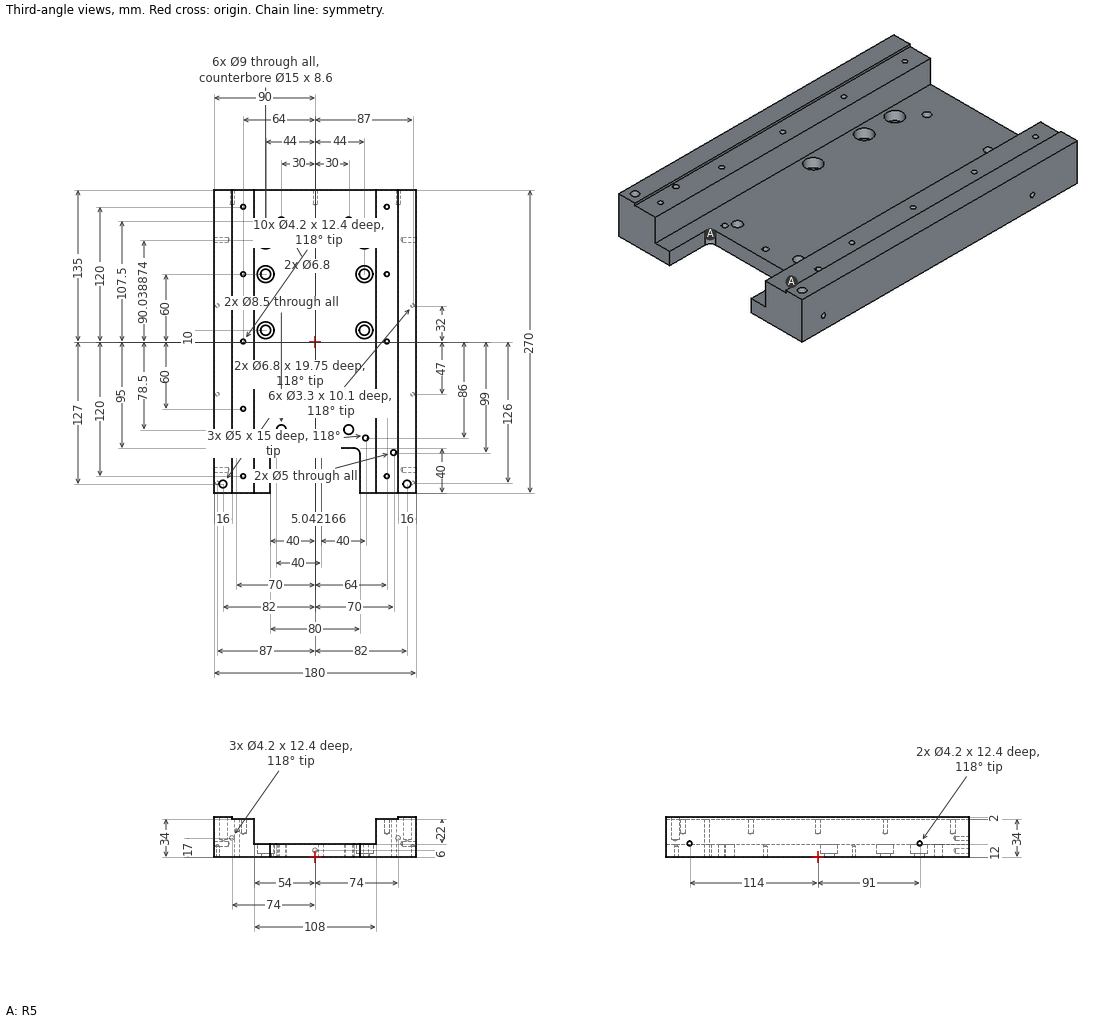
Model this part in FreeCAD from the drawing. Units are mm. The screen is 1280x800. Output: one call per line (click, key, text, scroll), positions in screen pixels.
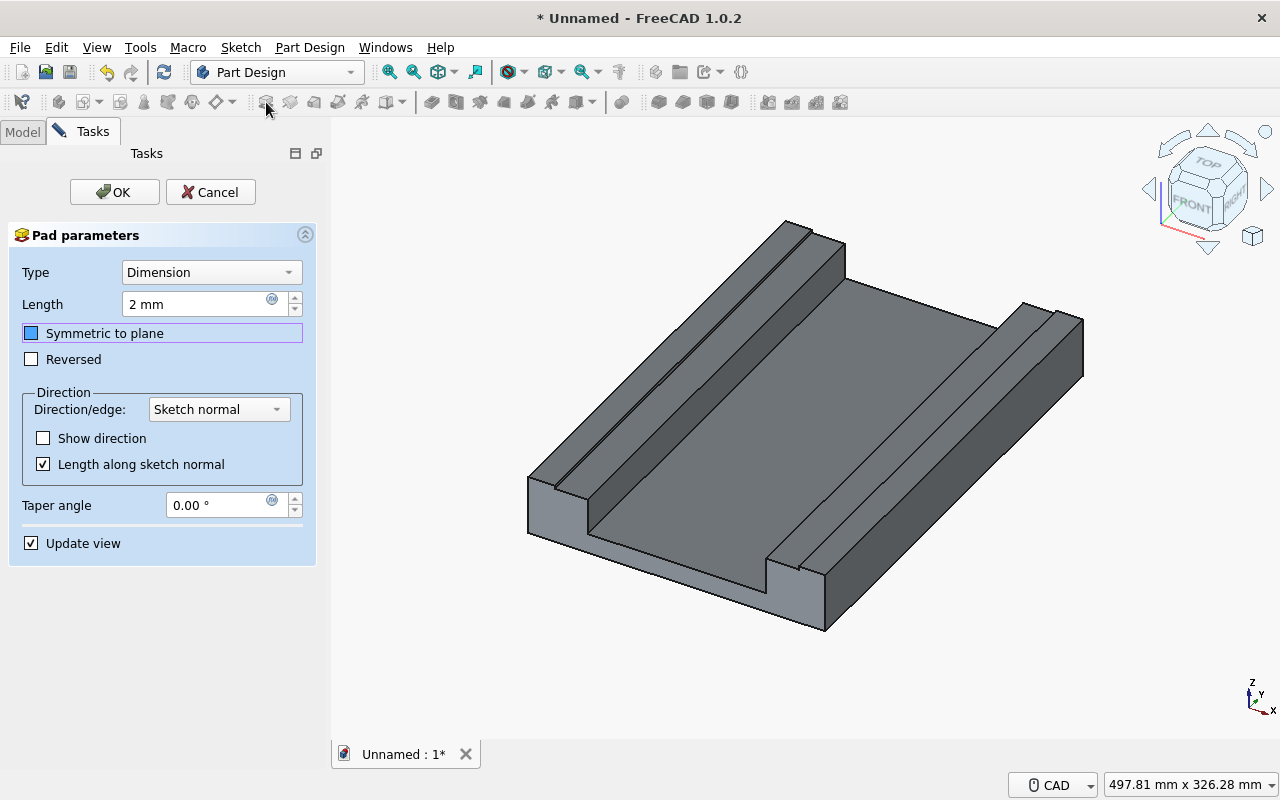
click(115, 192)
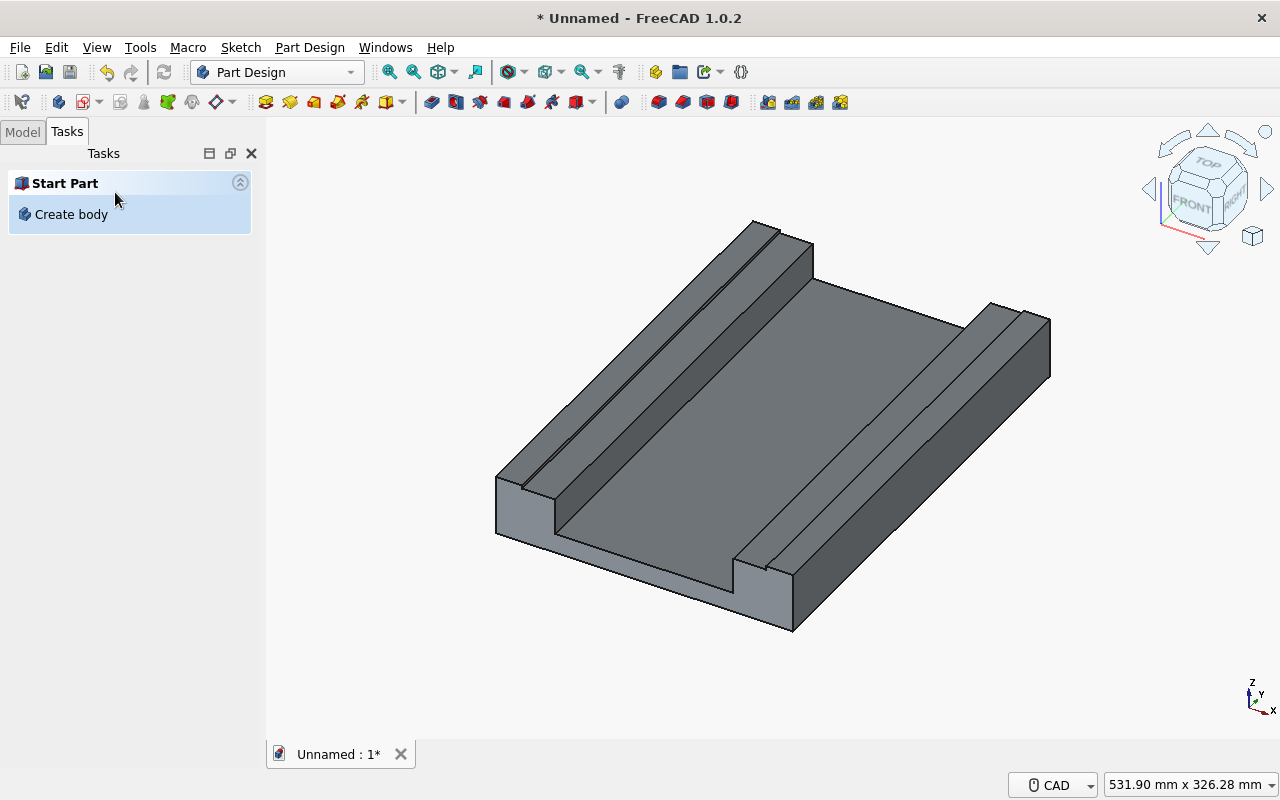
click(1019, 332)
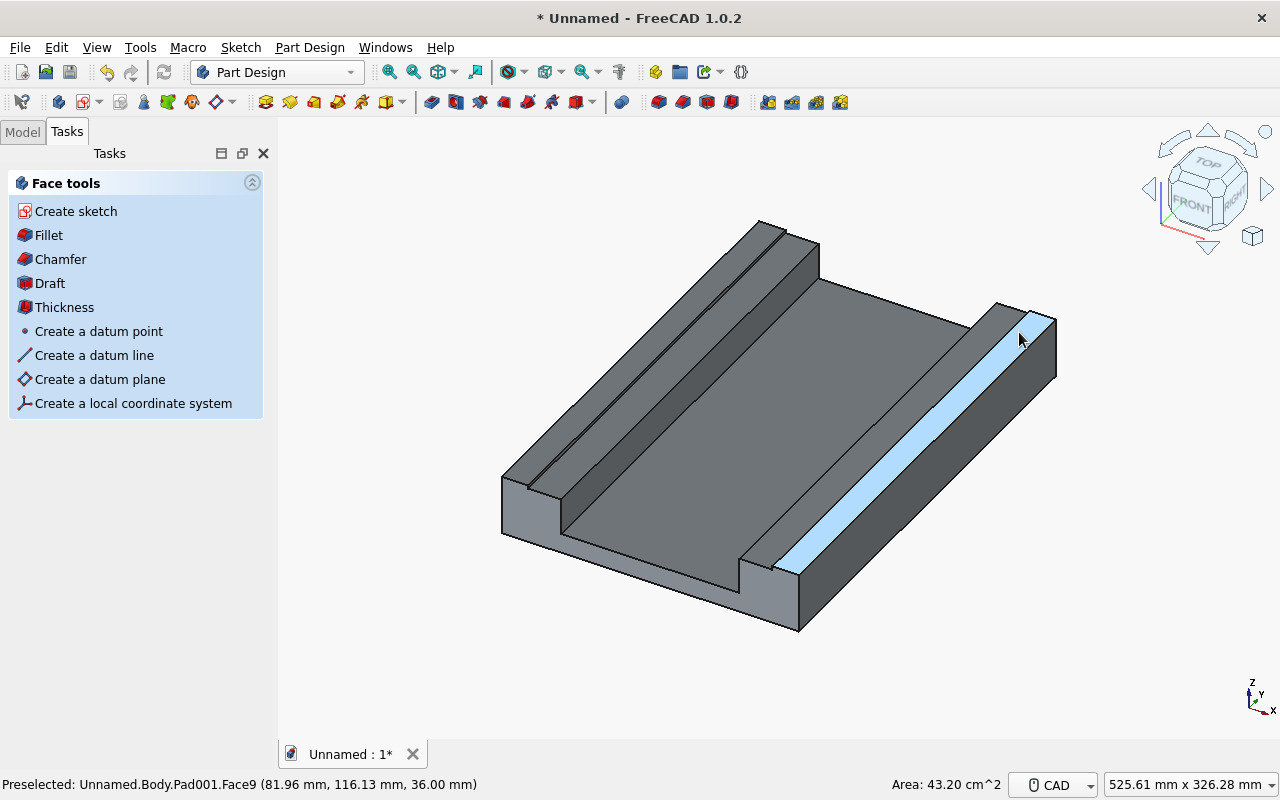
click(84, 102)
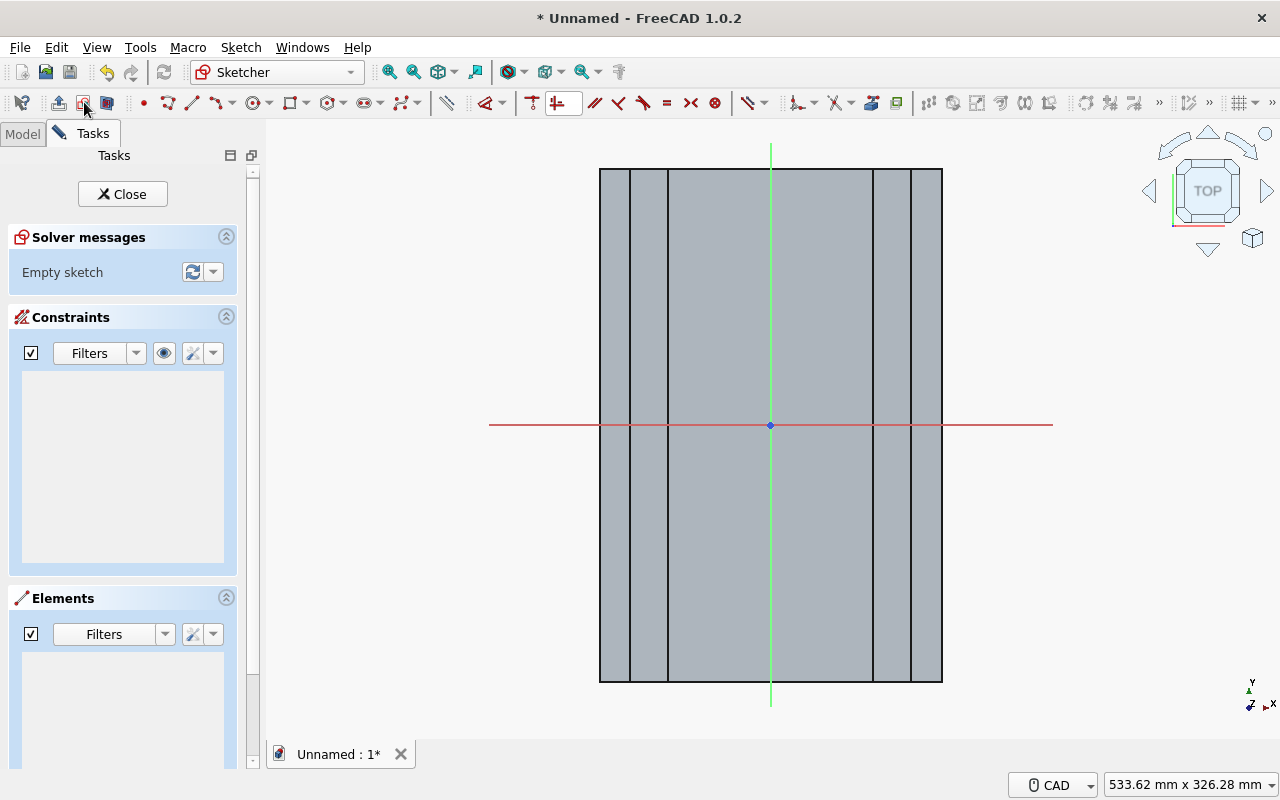
scroll(905, 711, up, 2)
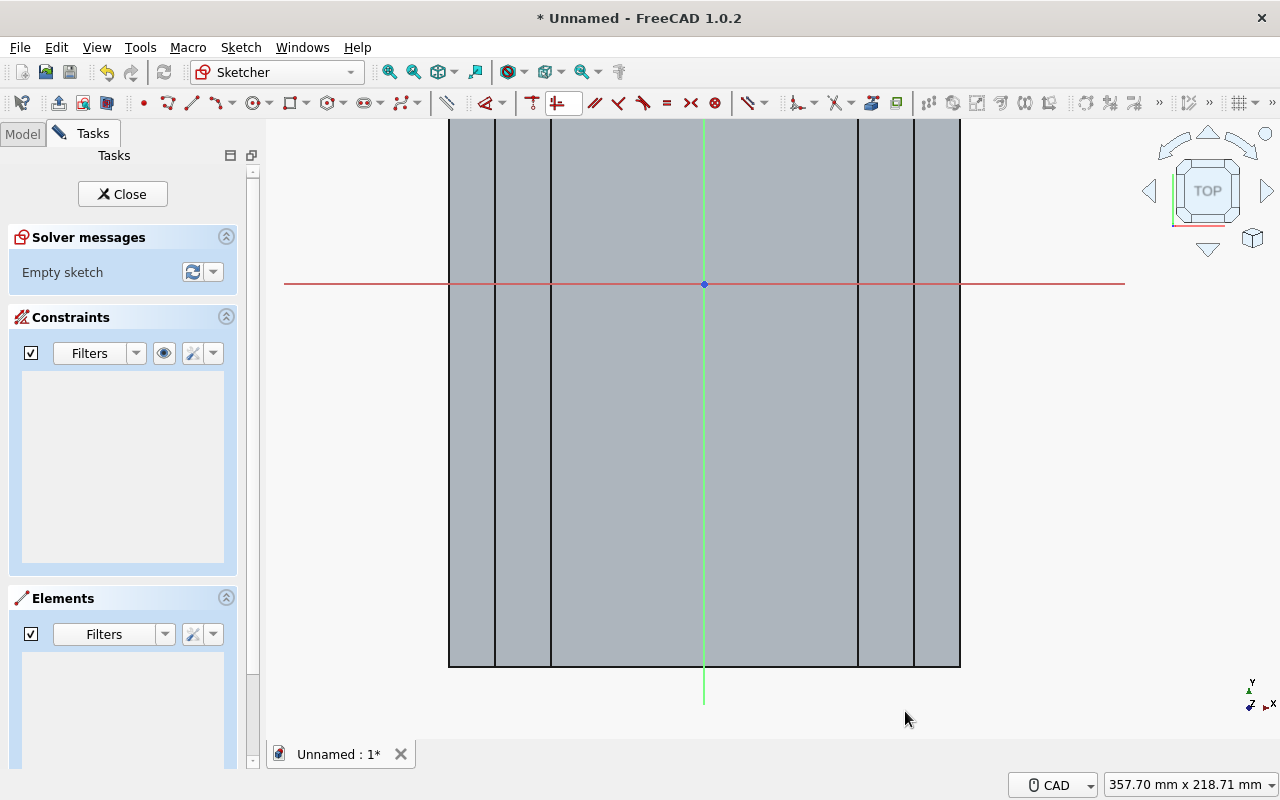
click(254, 104)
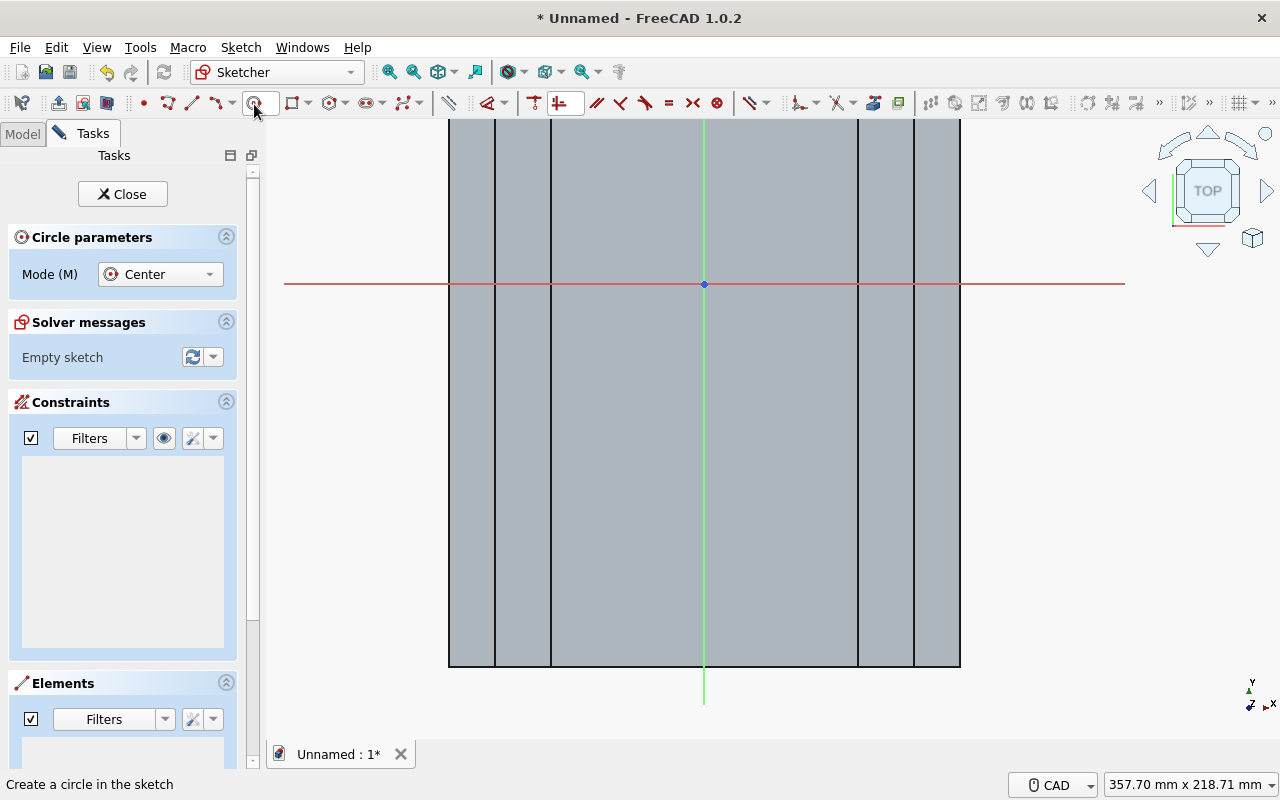
scroll(472, 644, up, 5)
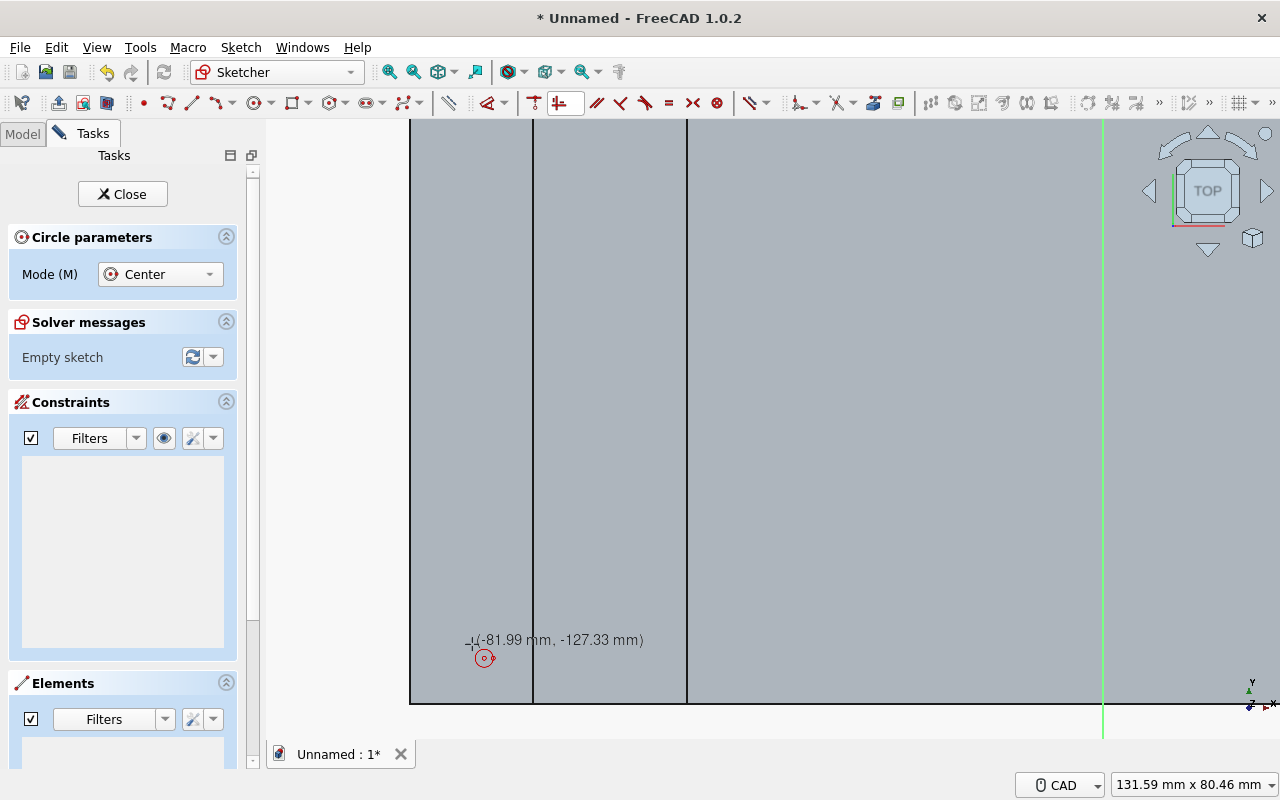
click(472, 643)
move(490, 624)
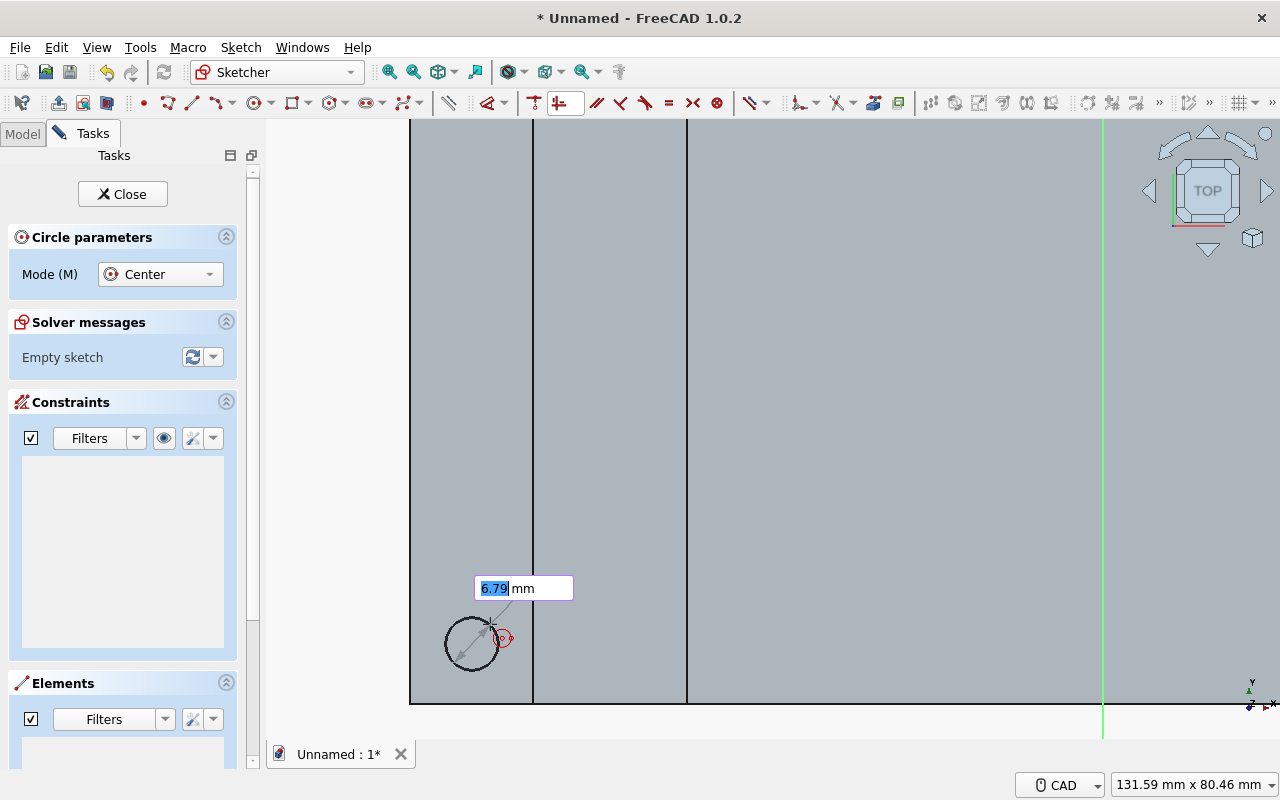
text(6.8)
key(Return)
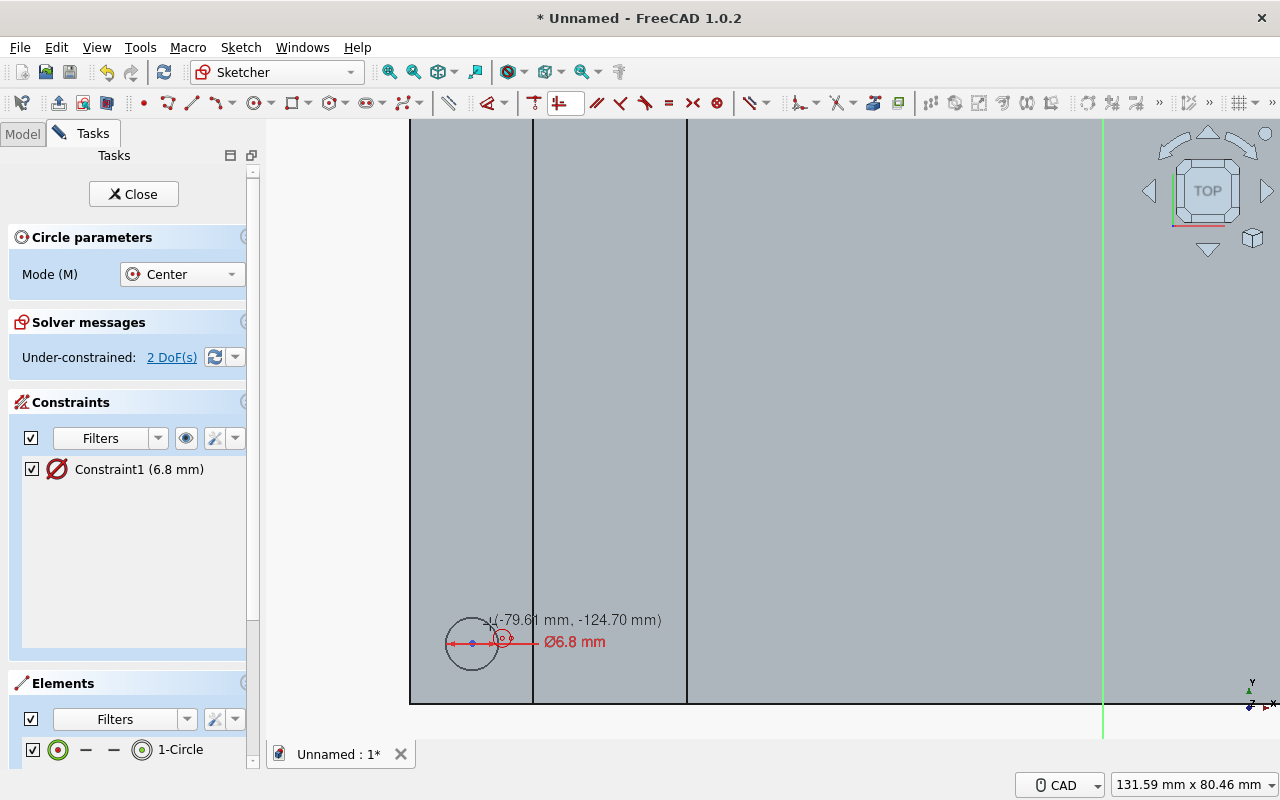
scroll(472, 582, down, 5)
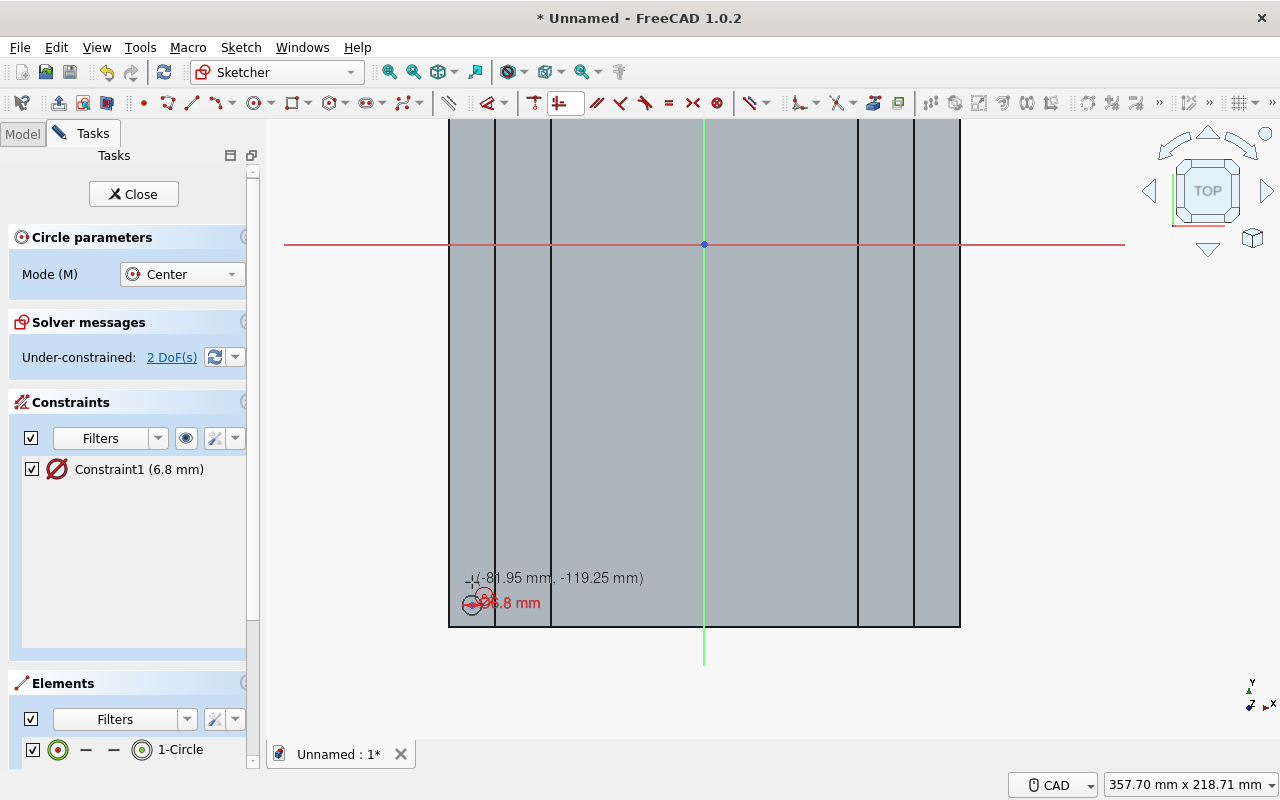
scroll(937, 605, up, 5)